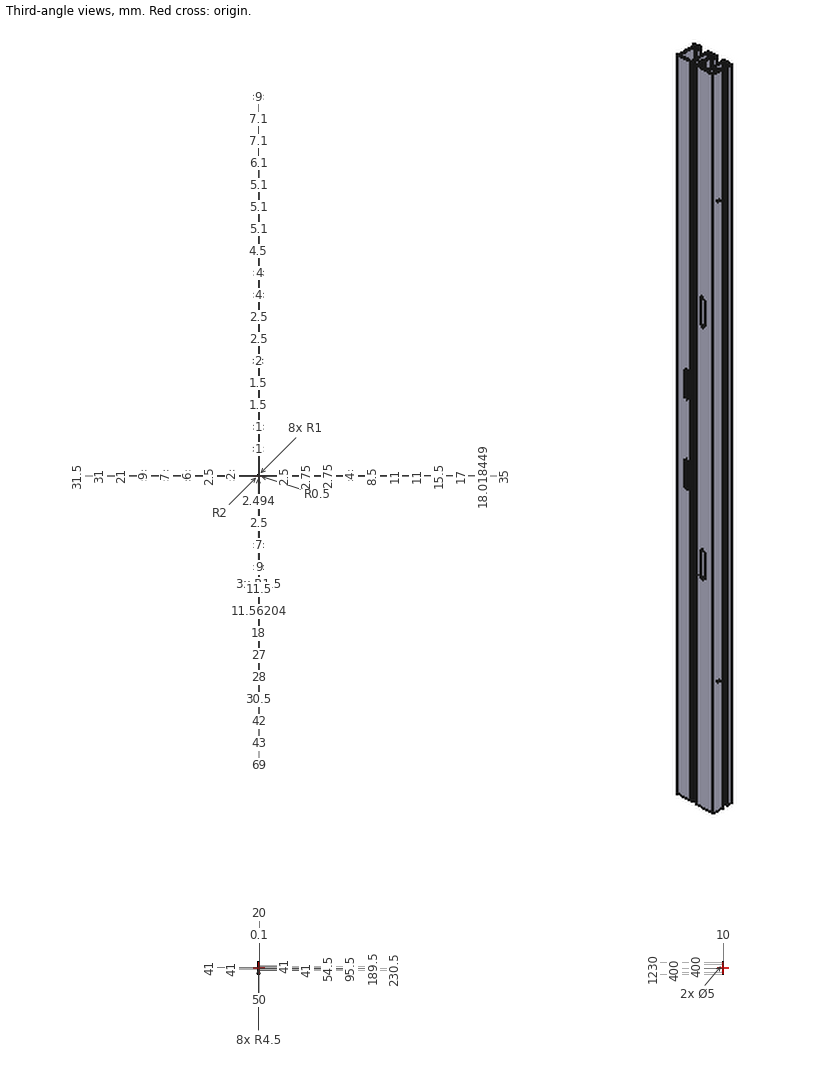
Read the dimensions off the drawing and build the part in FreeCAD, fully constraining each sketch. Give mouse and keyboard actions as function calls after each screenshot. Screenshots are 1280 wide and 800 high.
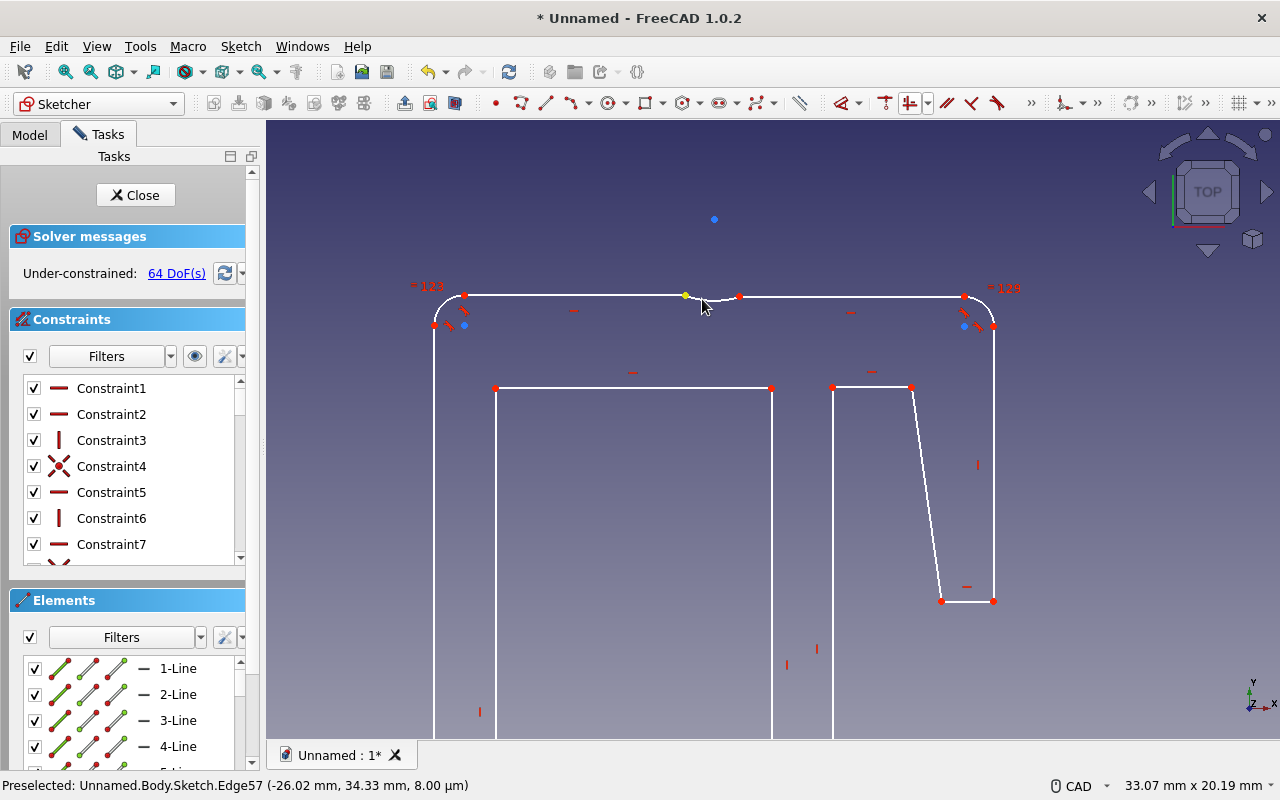
click(701, 300)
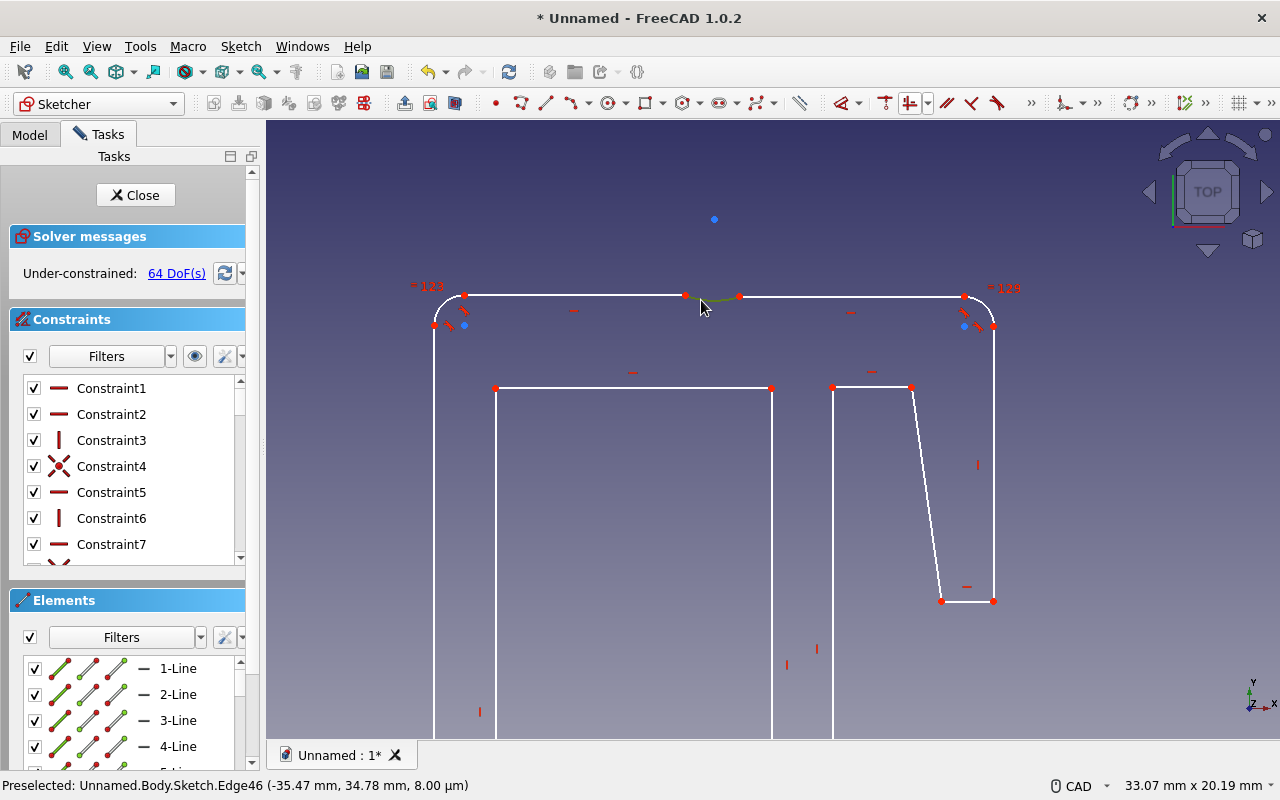
scroll(702, 299, down, 7)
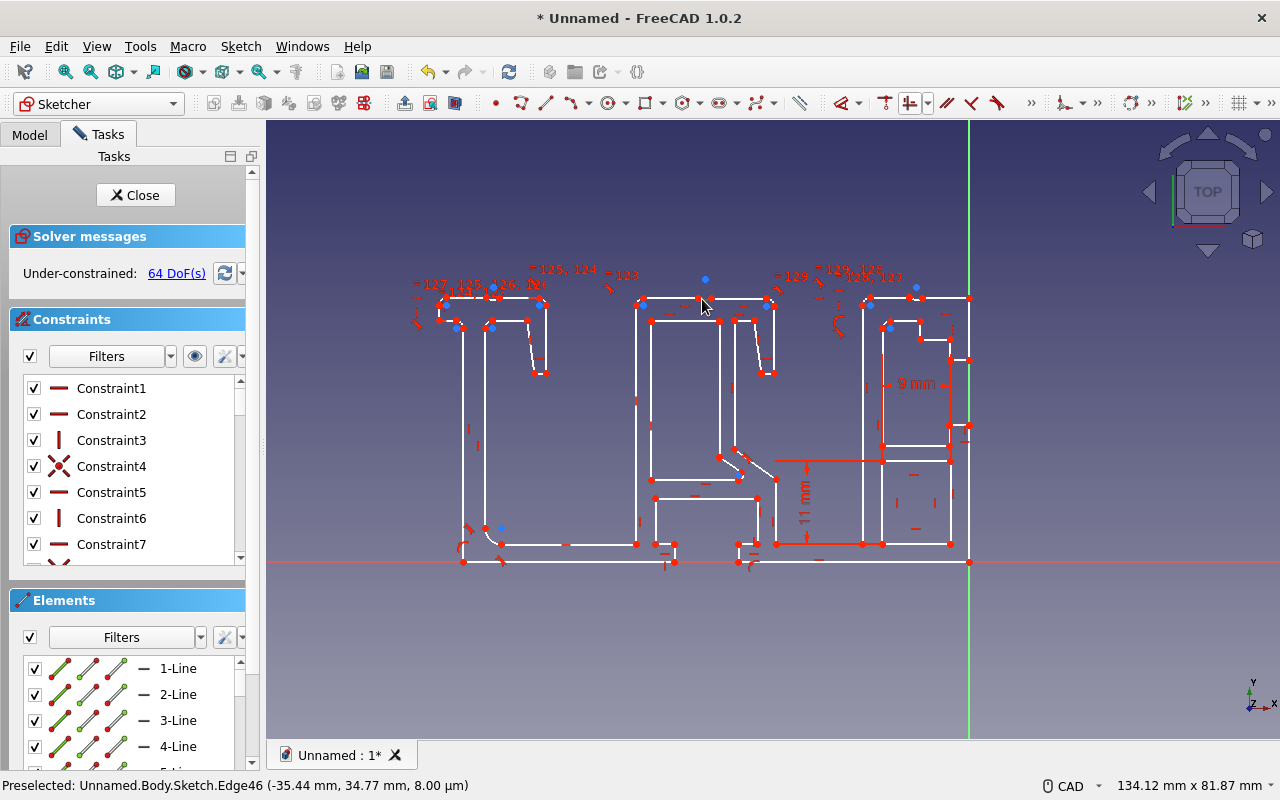
scroll(490, 299, up, 6)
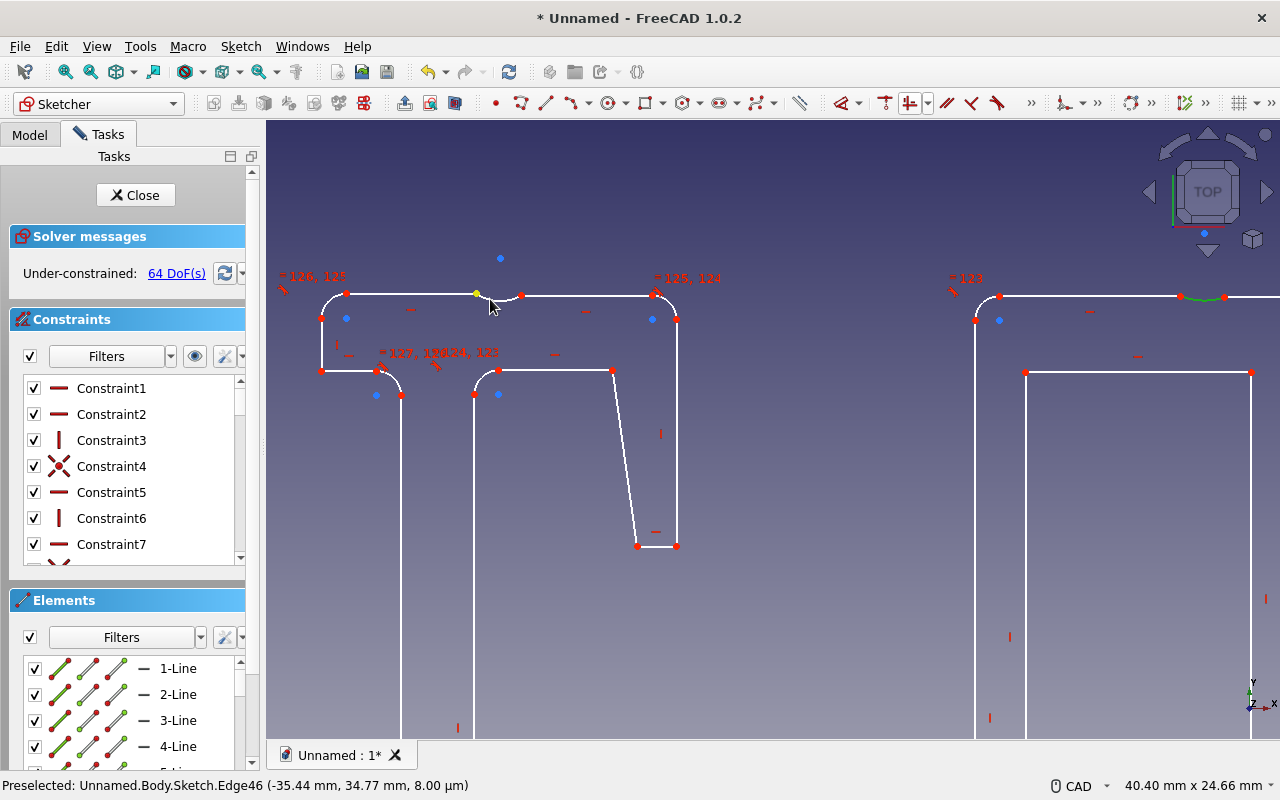
click(490, 300)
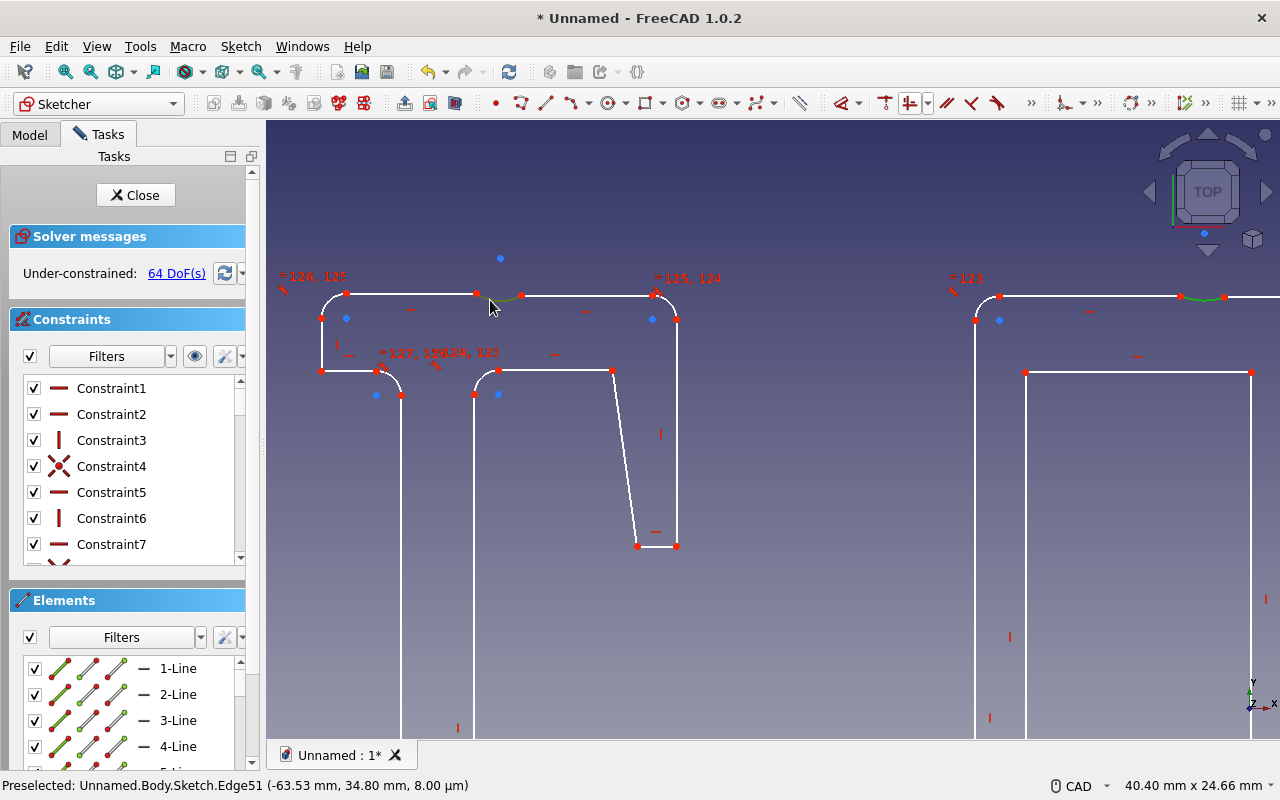
scroll(490, 299, down, 6)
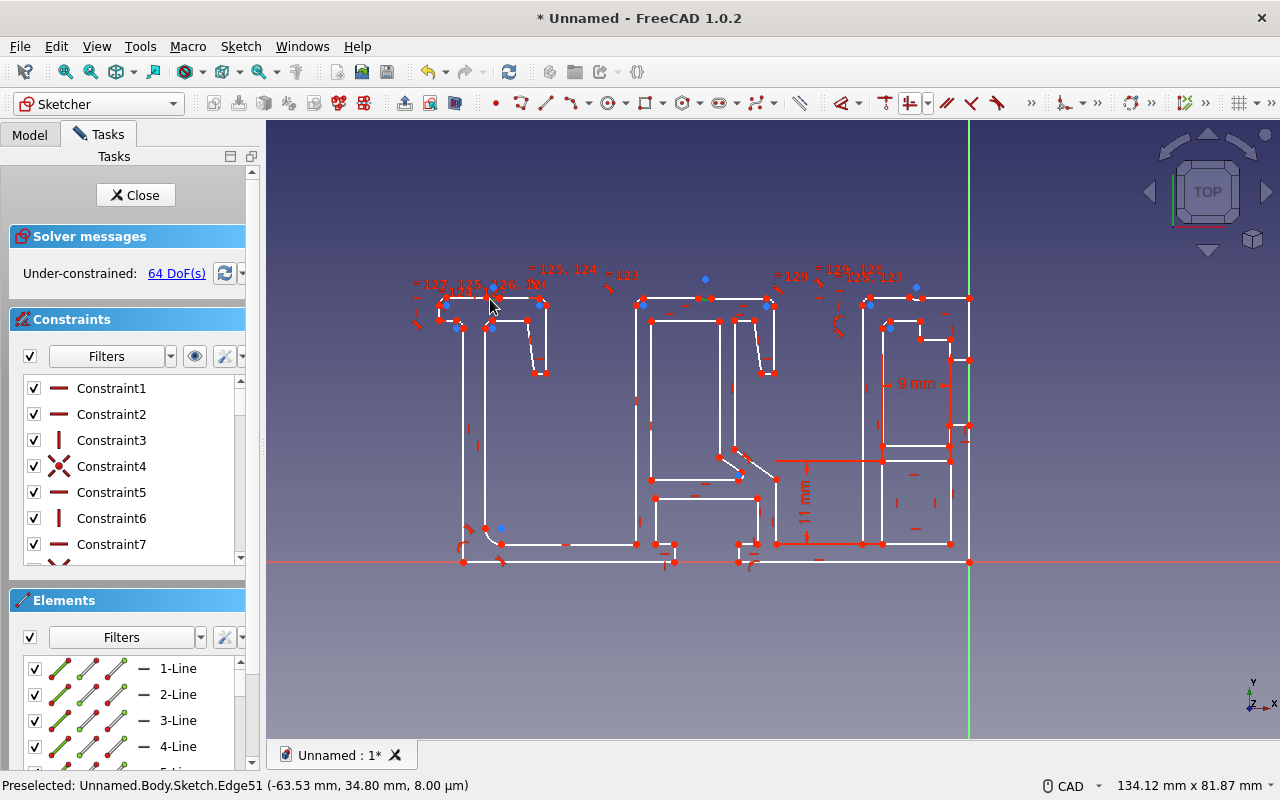
scroll(913, 299, up, 6)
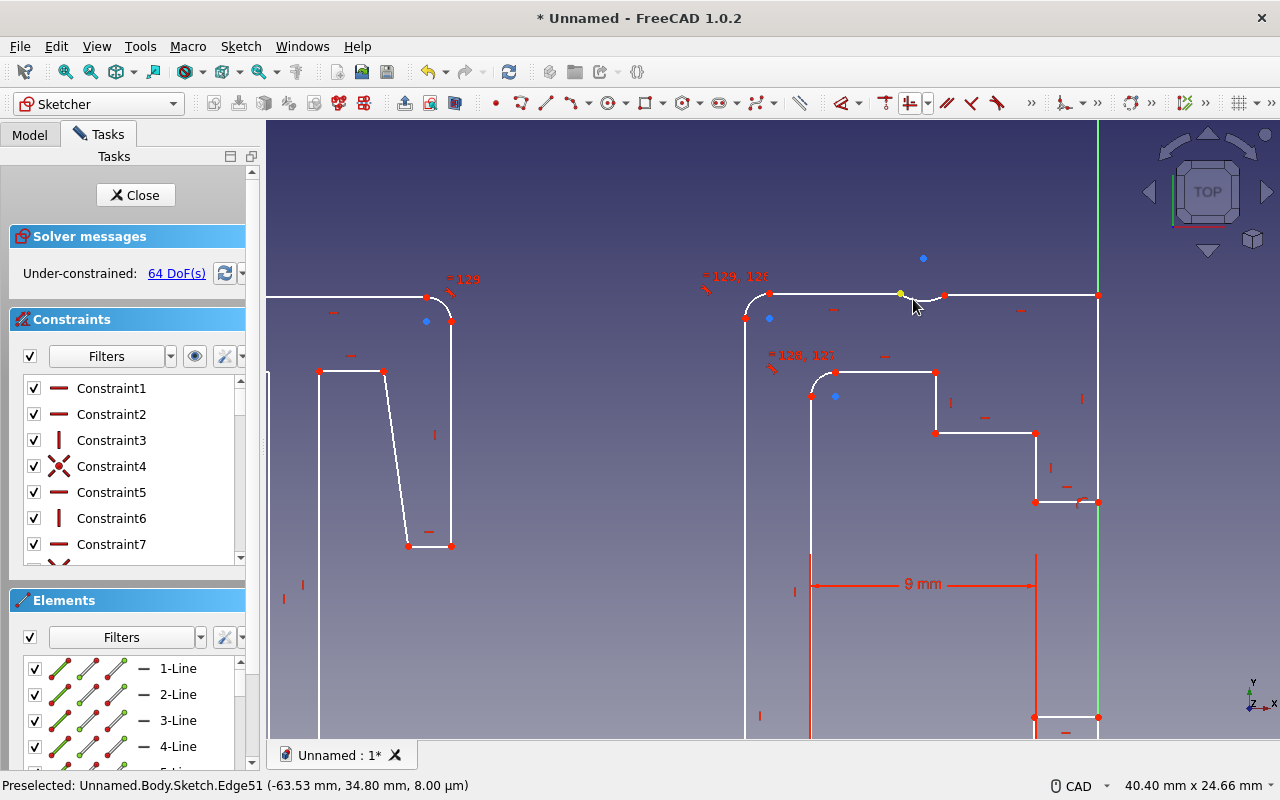
click(913, 300)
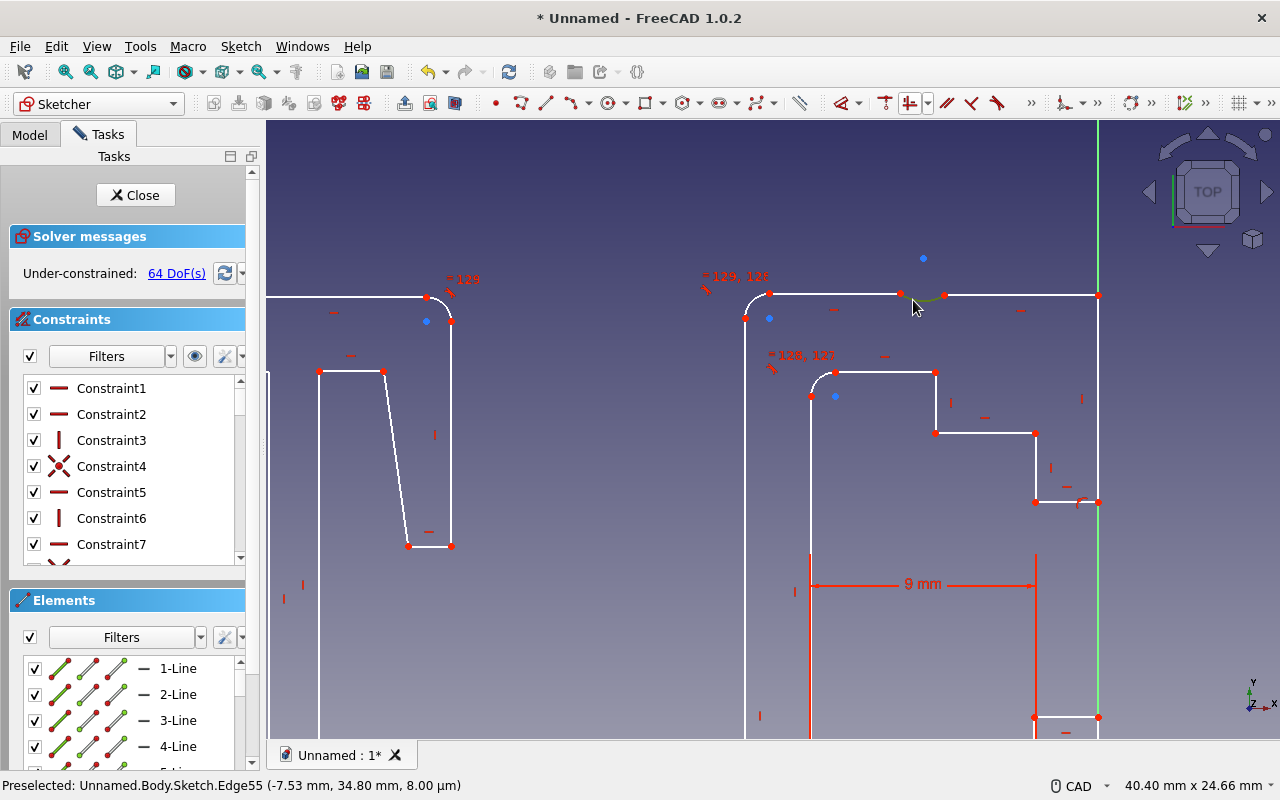
key(e)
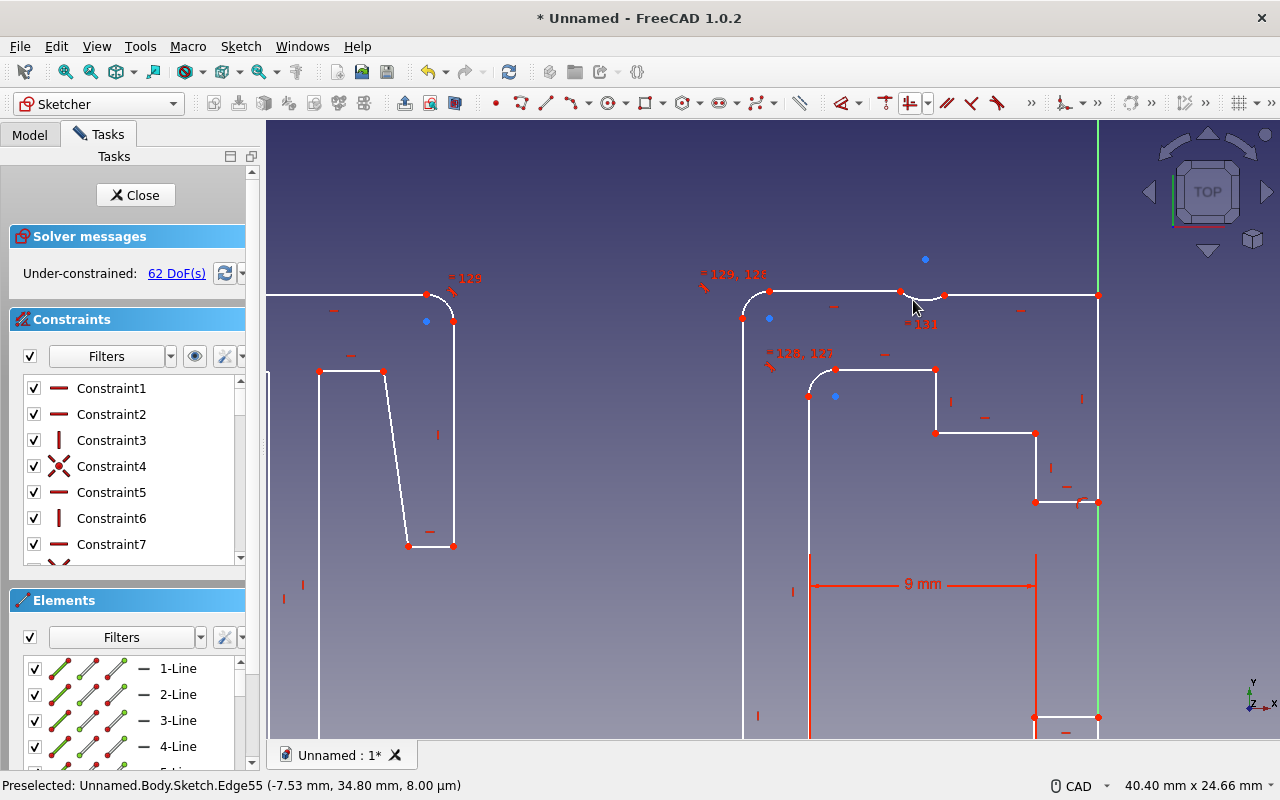
click(840, 104)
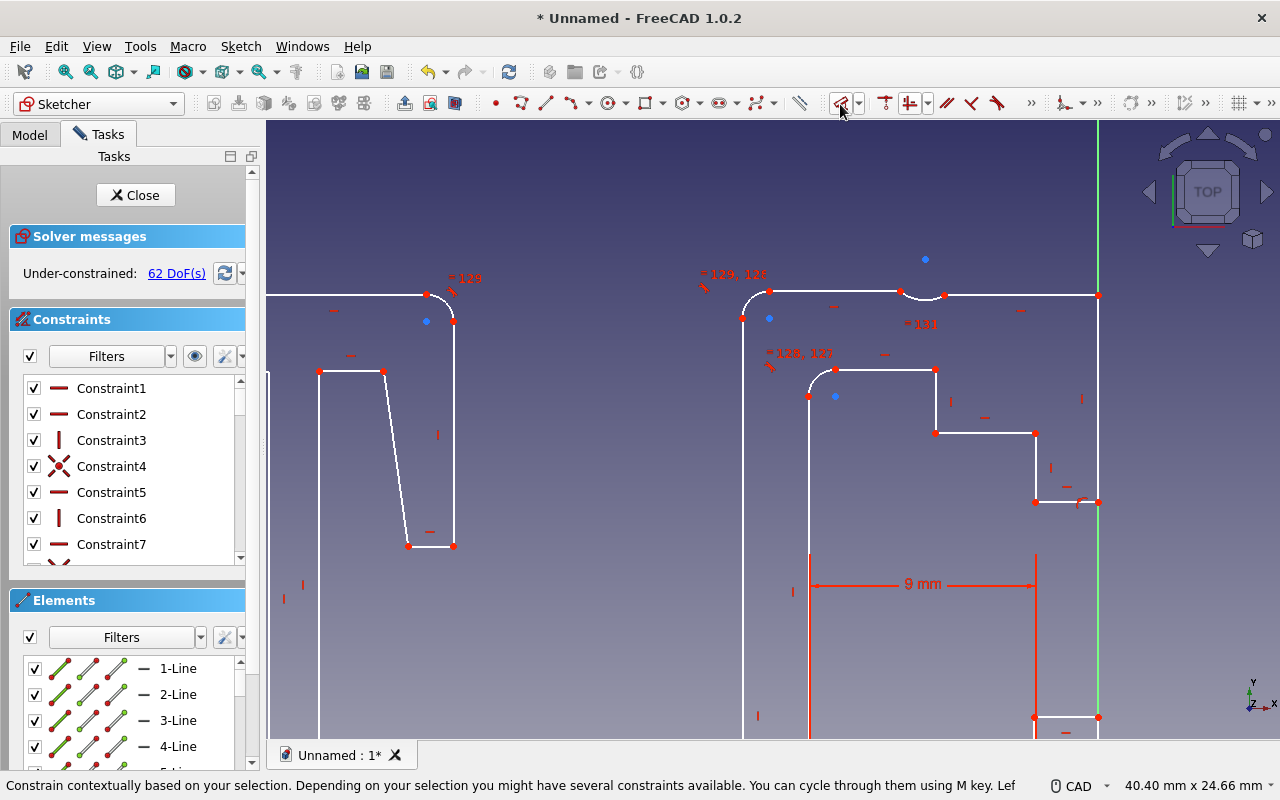
scroll(913, 299, down, 6)